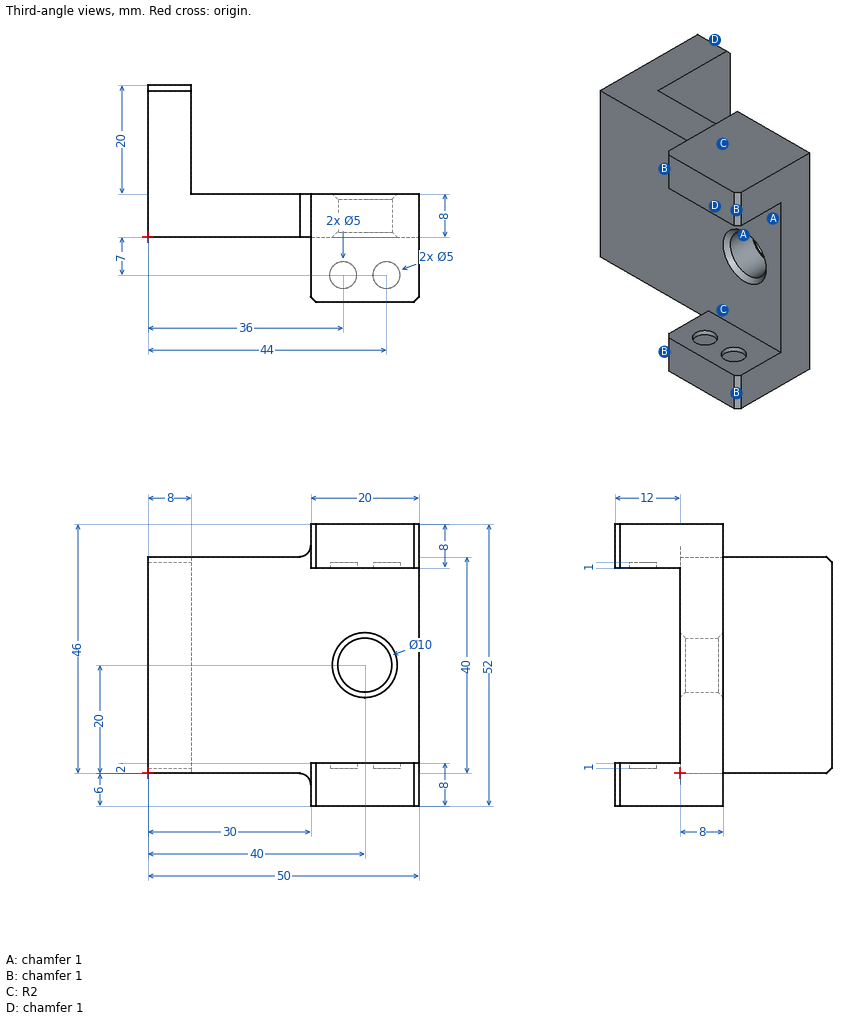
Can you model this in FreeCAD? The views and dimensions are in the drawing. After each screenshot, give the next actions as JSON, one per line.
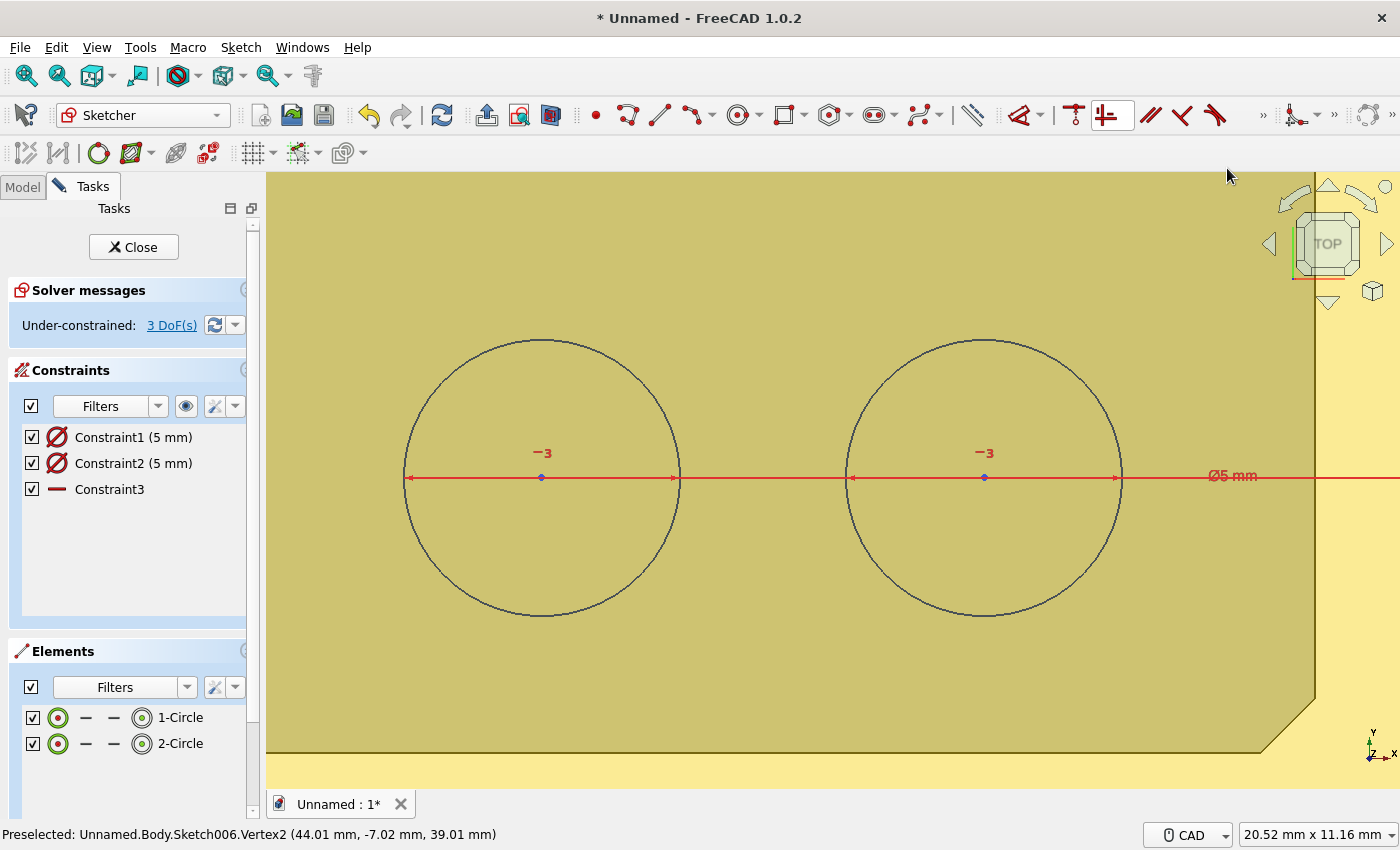
{"action": "left_click", "coordinate": [1020, 116]}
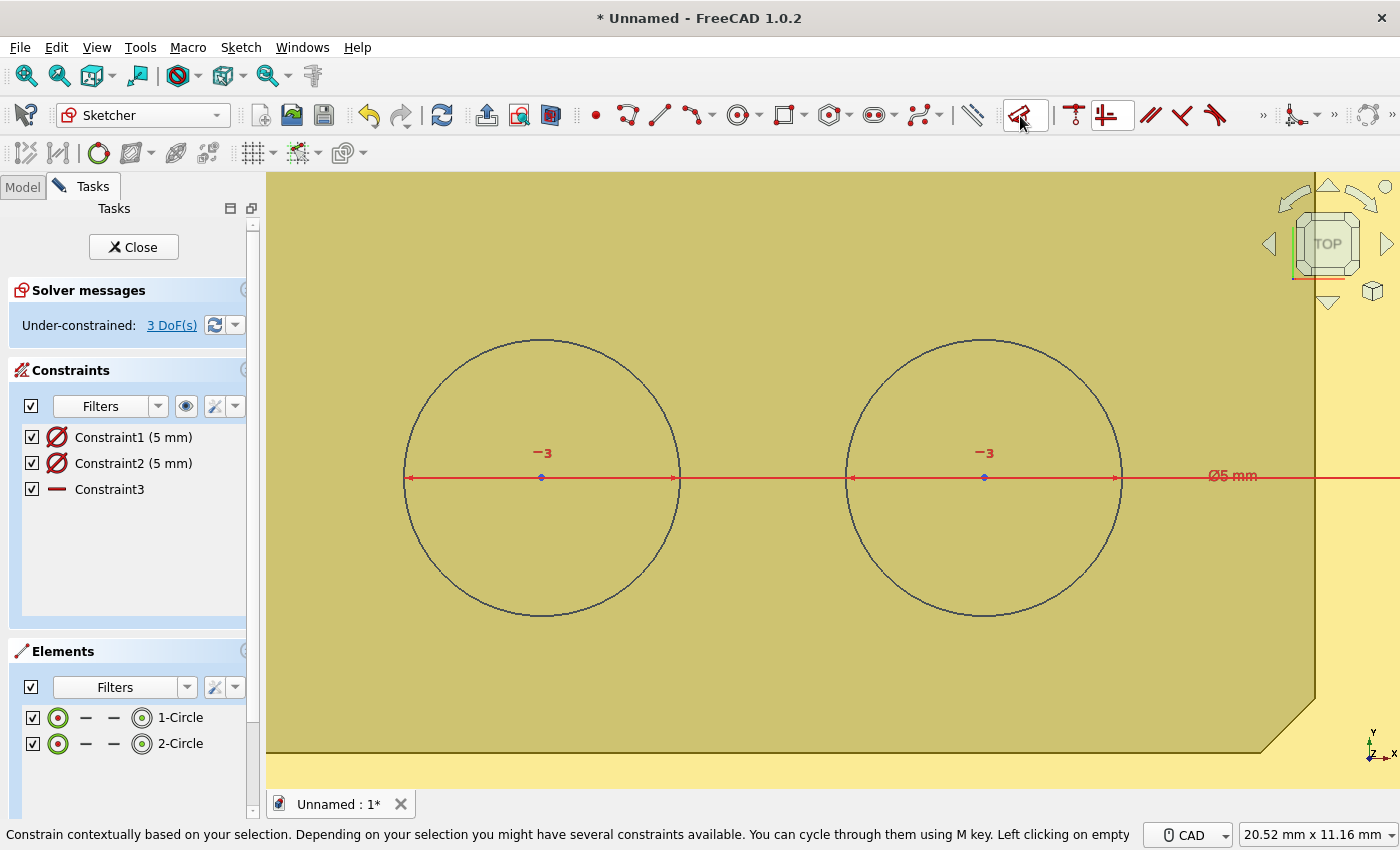
{"action": "left_click", "coordinate": [542, 478]}
{"action": "left_click", "coordinate": [576, 275]}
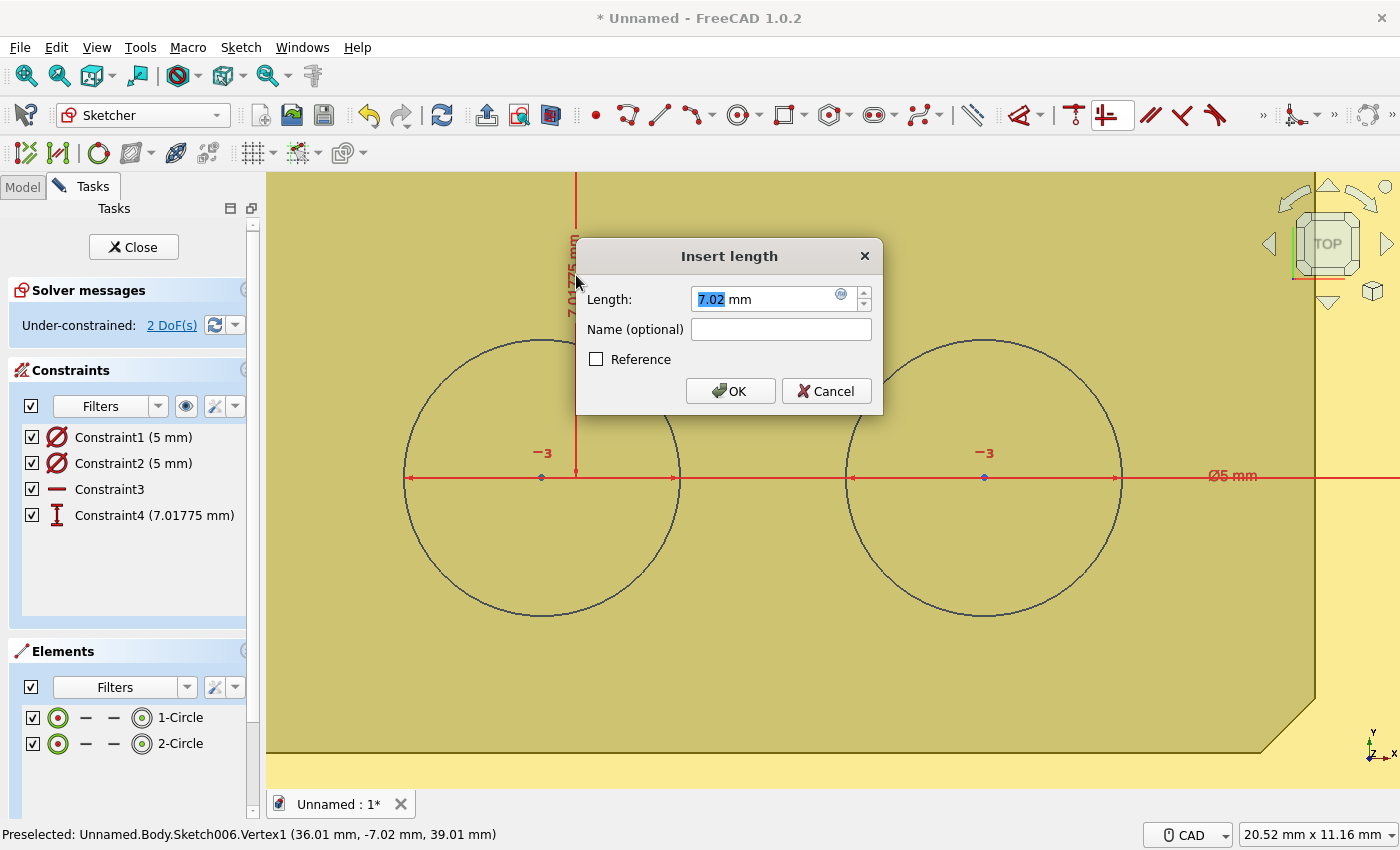
{"action": "type", "text": "7"}
{"action": "key", "text": "Return"}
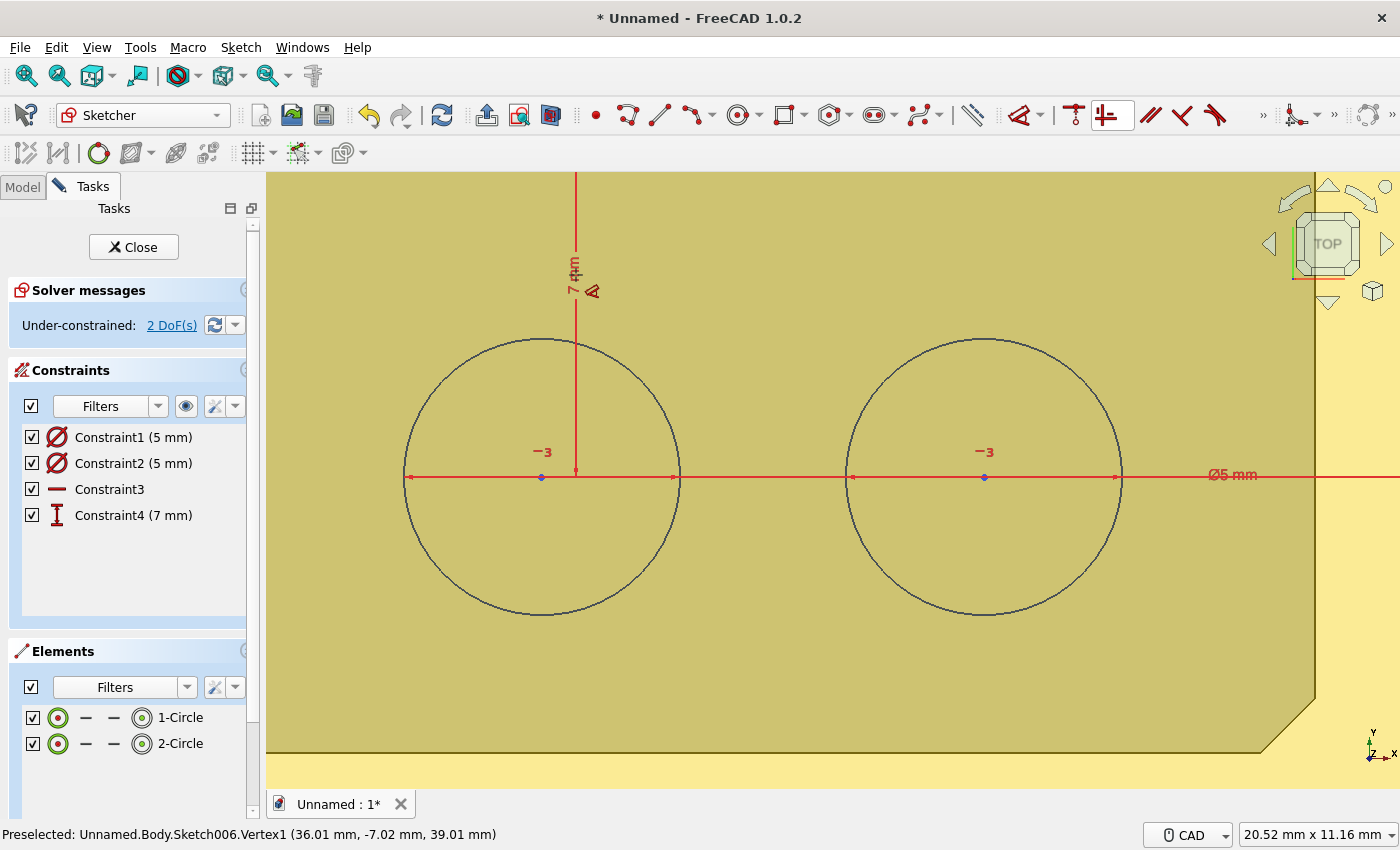
{"action": "left_click", "coordinate": [542, 477]}
{"action": "left_click", "coordinate": [361, 511]}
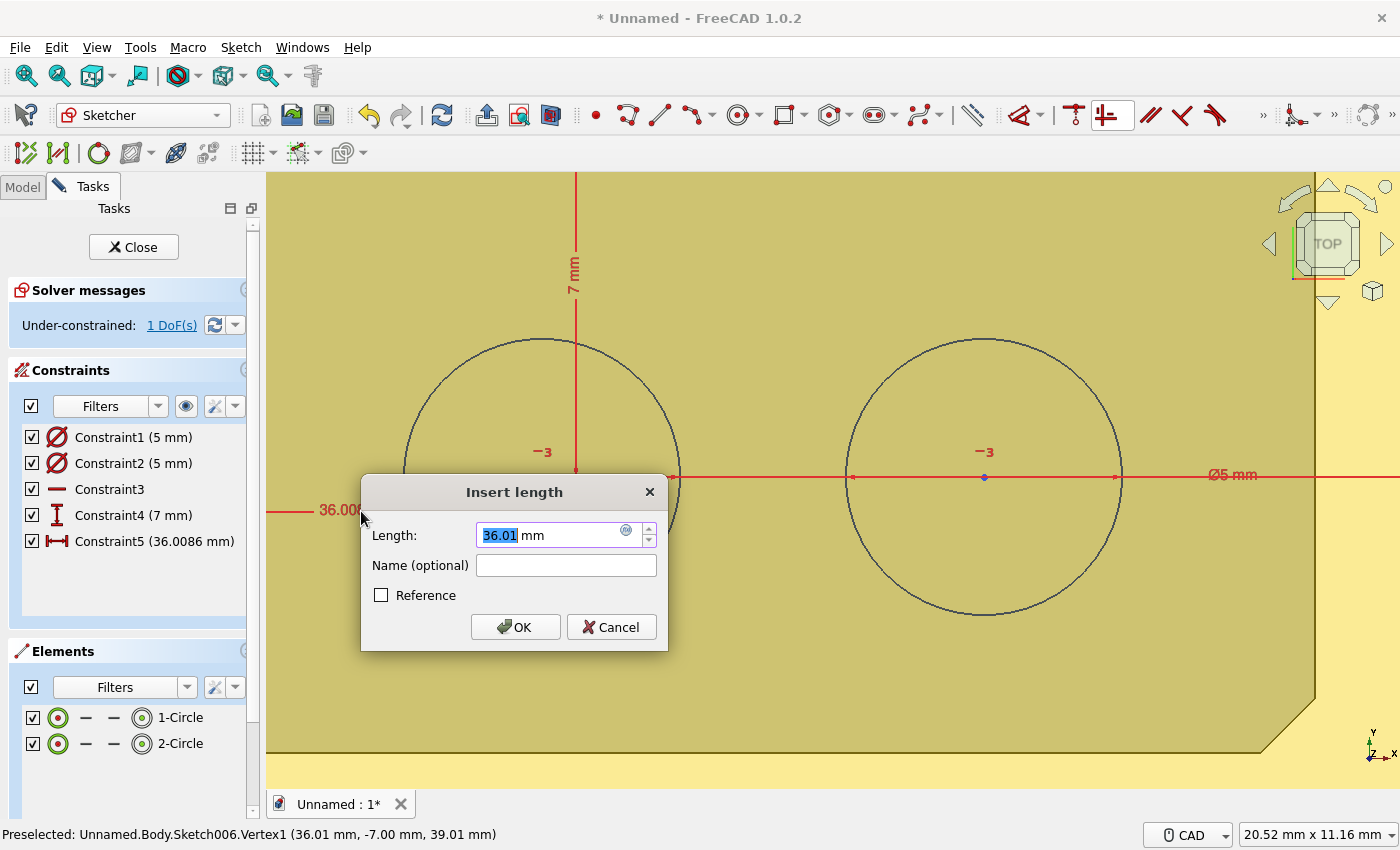
{"action": "type", "text": "36"}
{"action": "key", "text": "Return"}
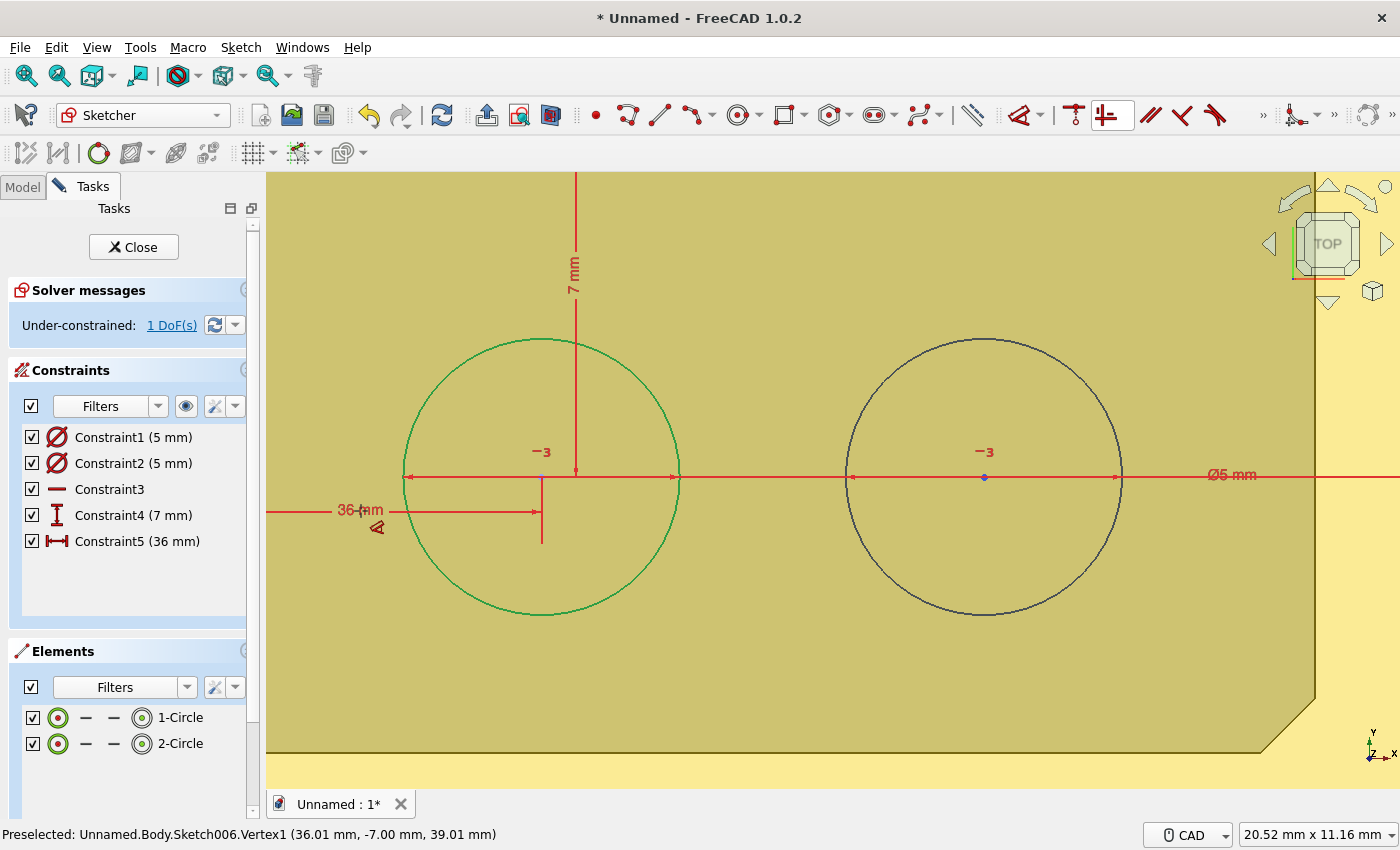
{"action": "left_click", "coordinate": [984, 477]}
{"action": "left_click", "coordinate": [639, 511]}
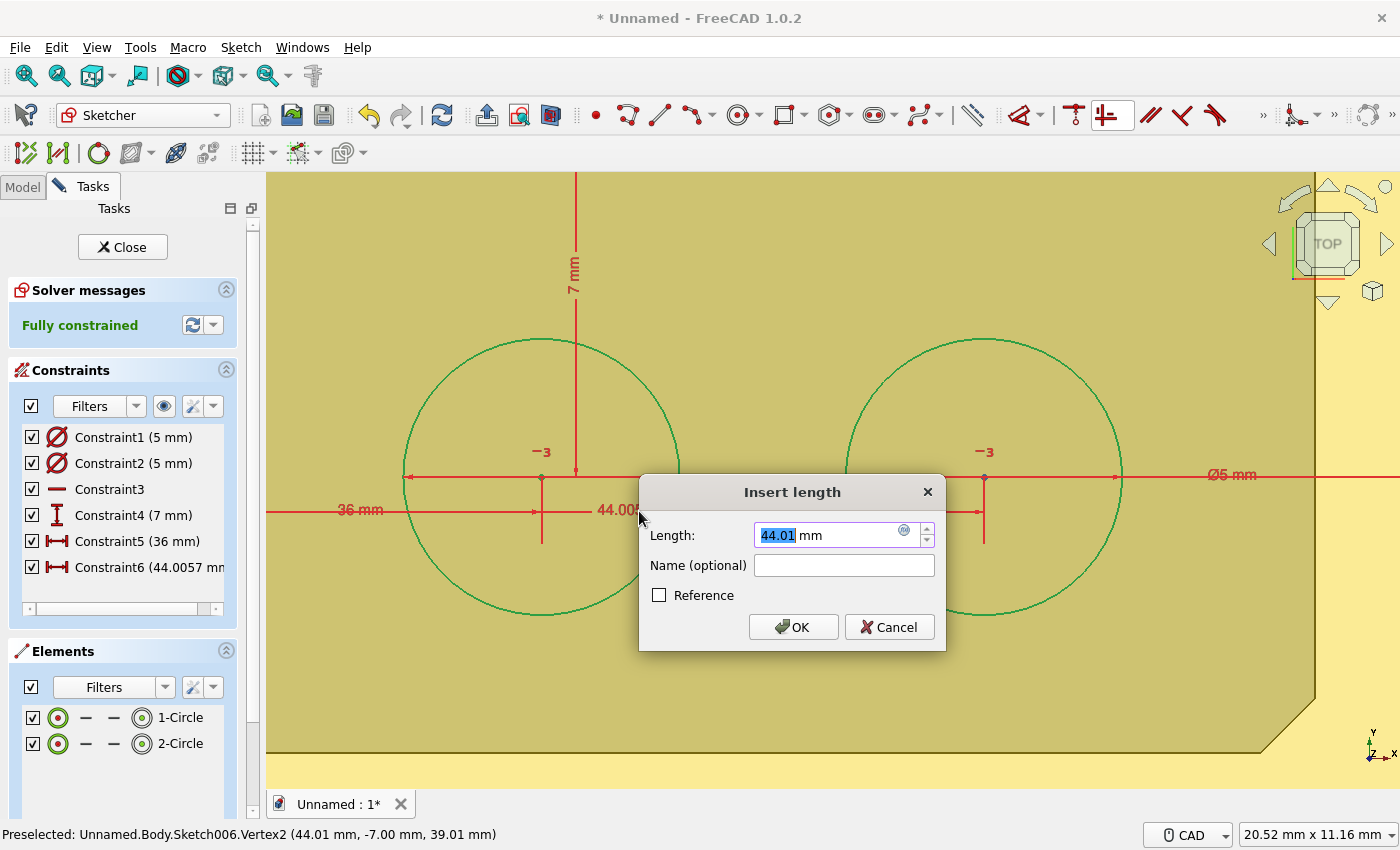
{"action": "type", "text": "44"}
{"action": "key", "text": "Return"}
{"action": "key", "text": "Escape"}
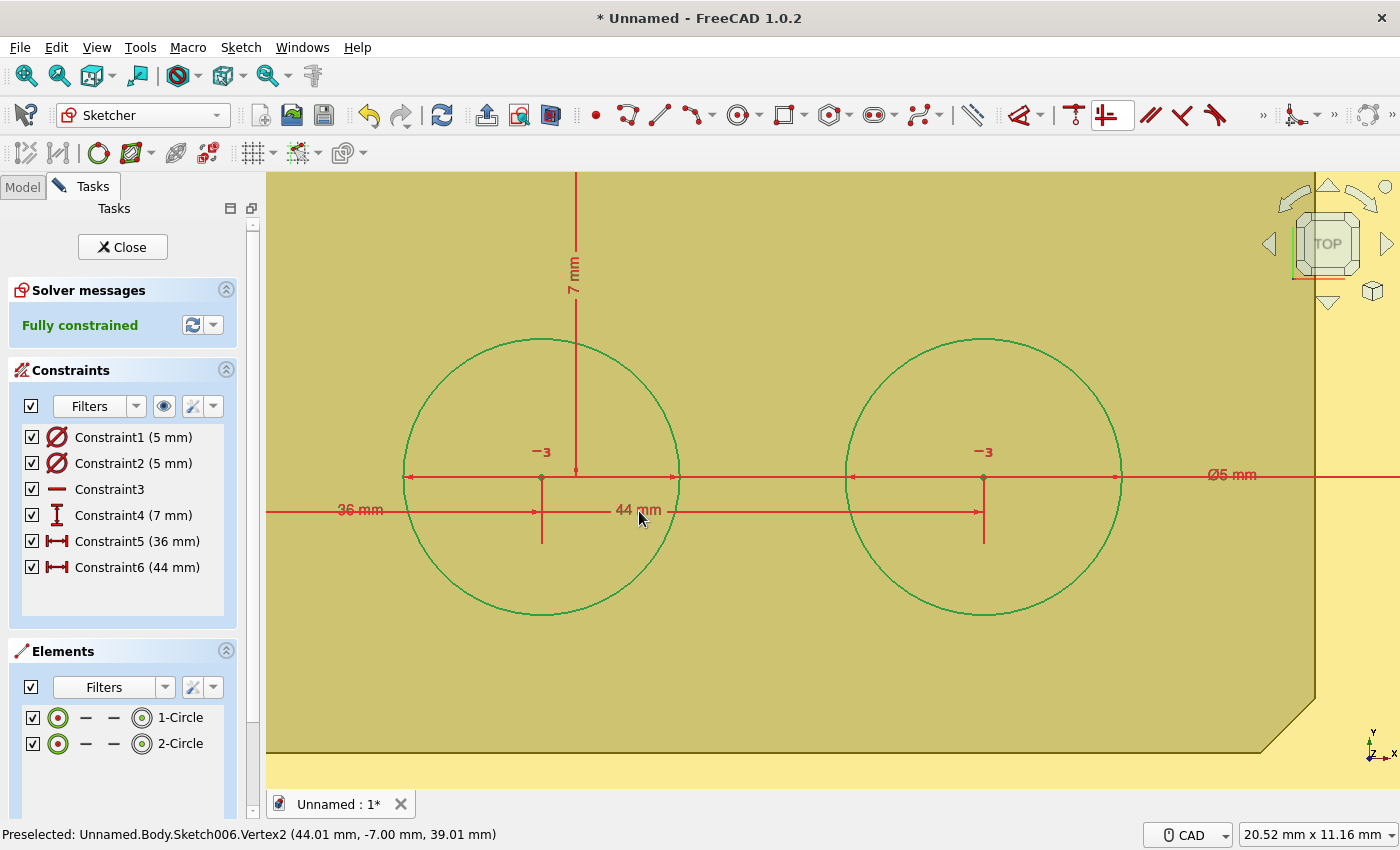
{"action": "left_click", "coordinate": [123, 247]}